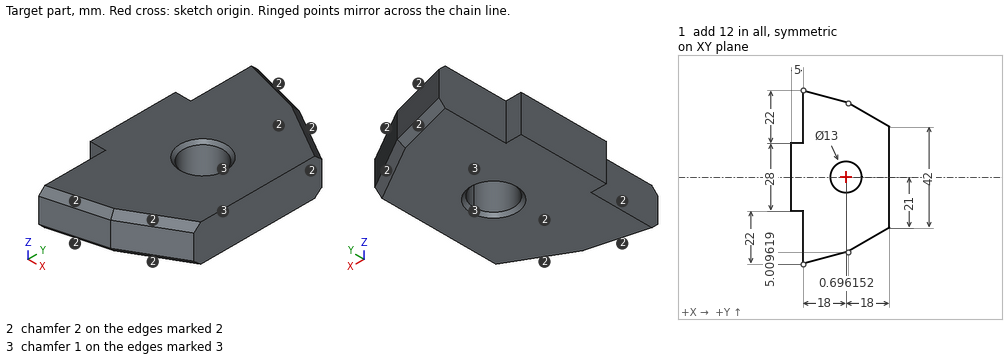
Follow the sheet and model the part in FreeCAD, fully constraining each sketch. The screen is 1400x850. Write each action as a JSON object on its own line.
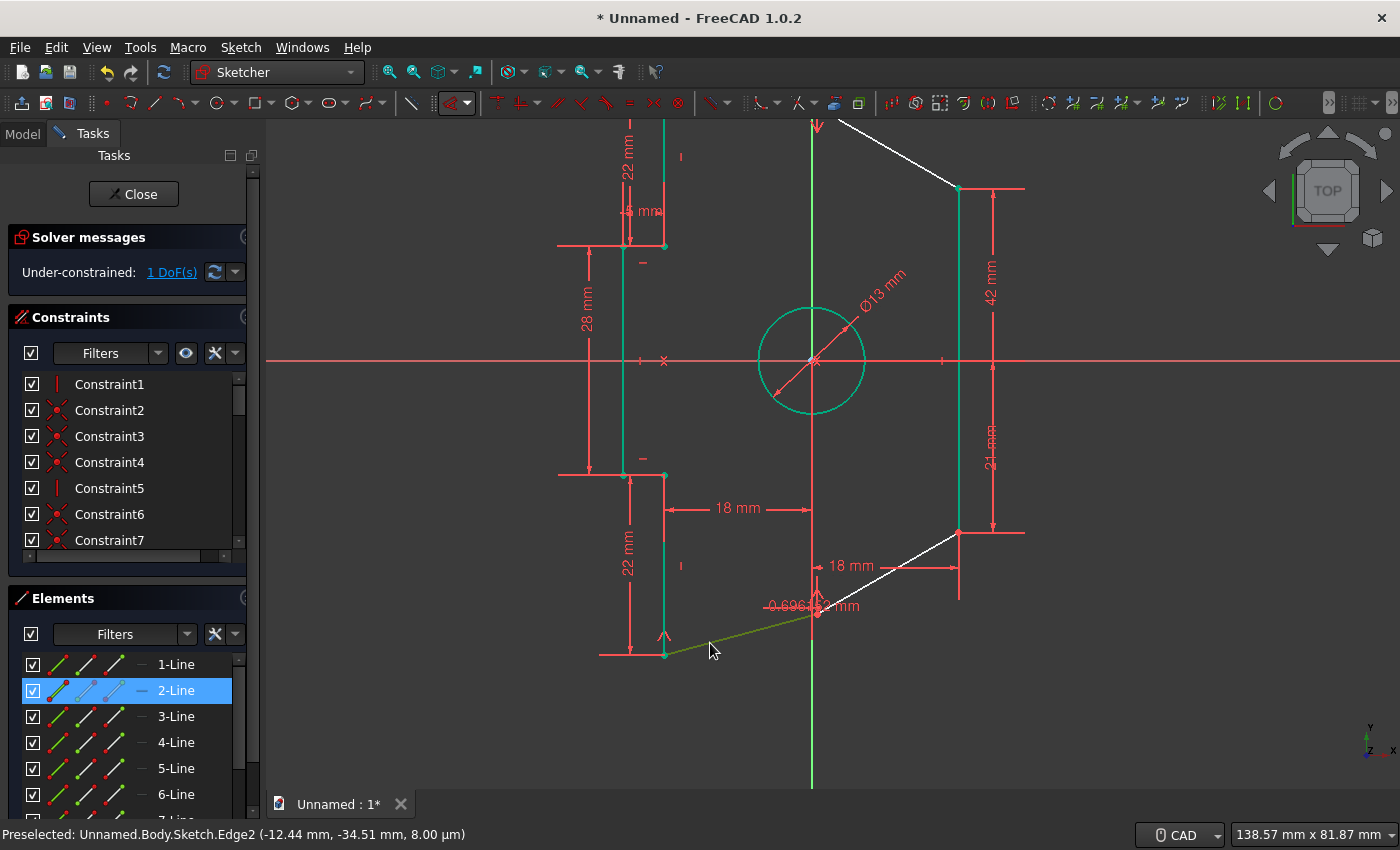
{"action": "left_click", "coordinate": [470, 104]}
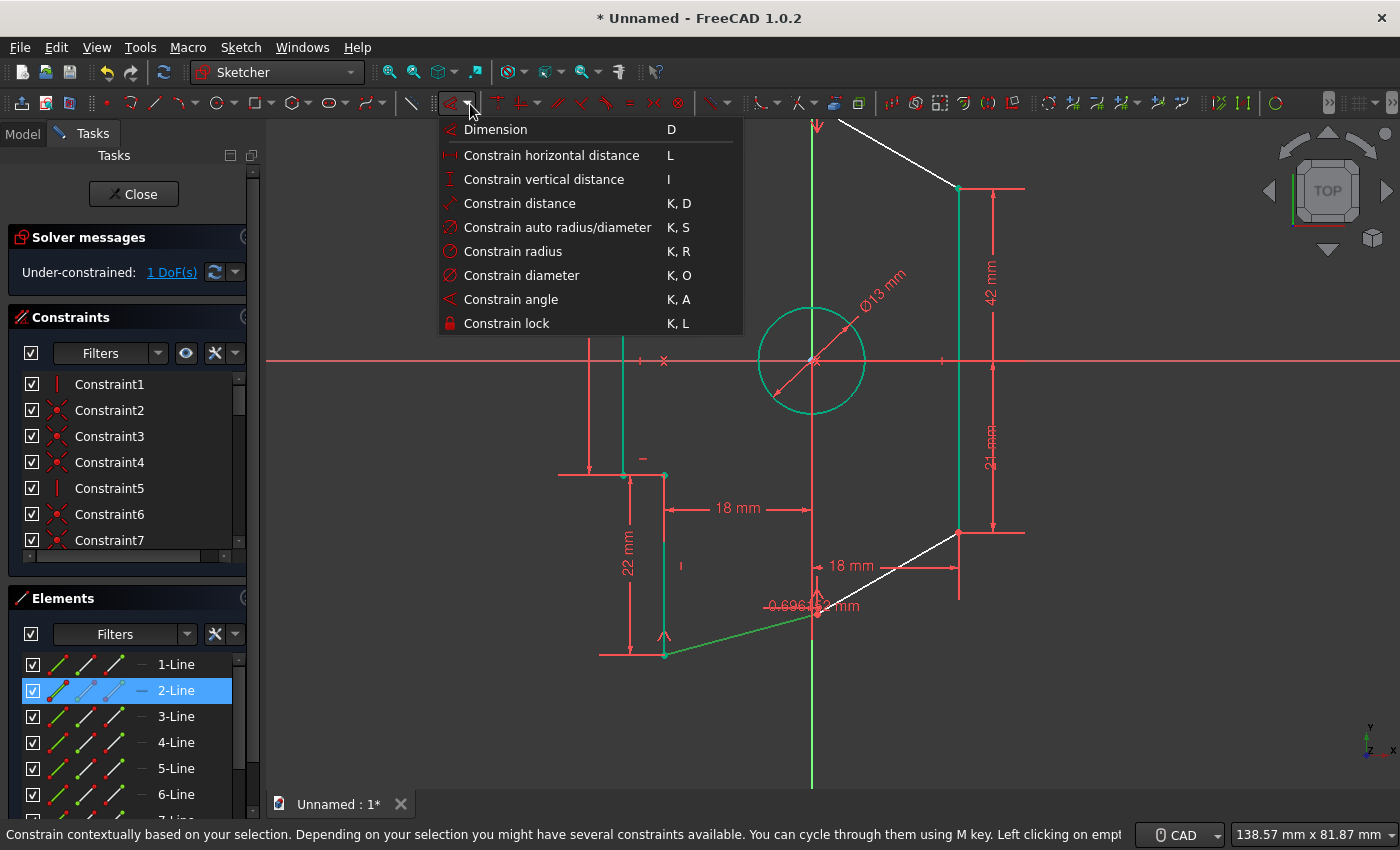
{"action": "left_click", "coordinate": [591, 179]}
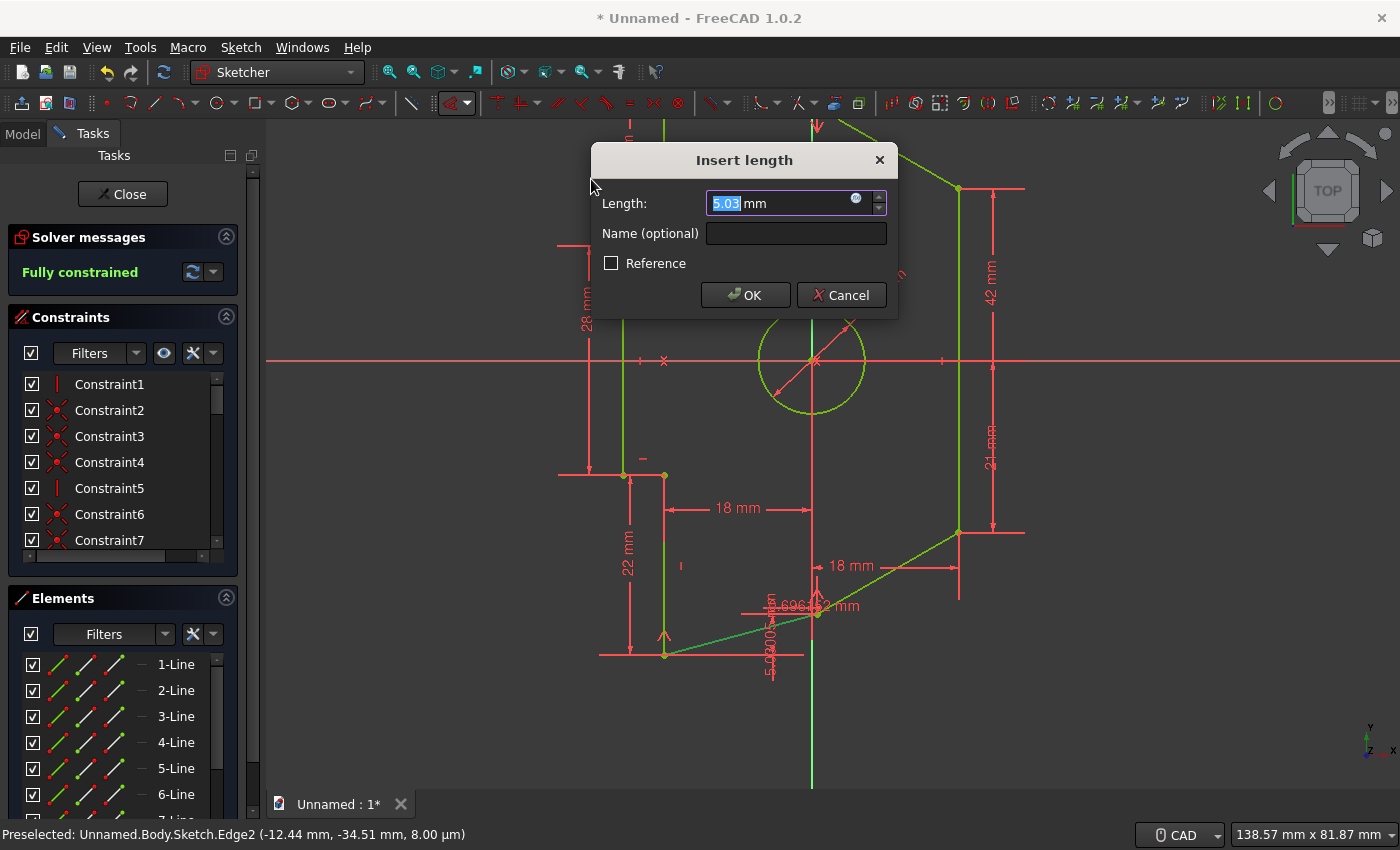
{"action": "type", "text": "5.009619"}
{"action": "key", "text": "Return"}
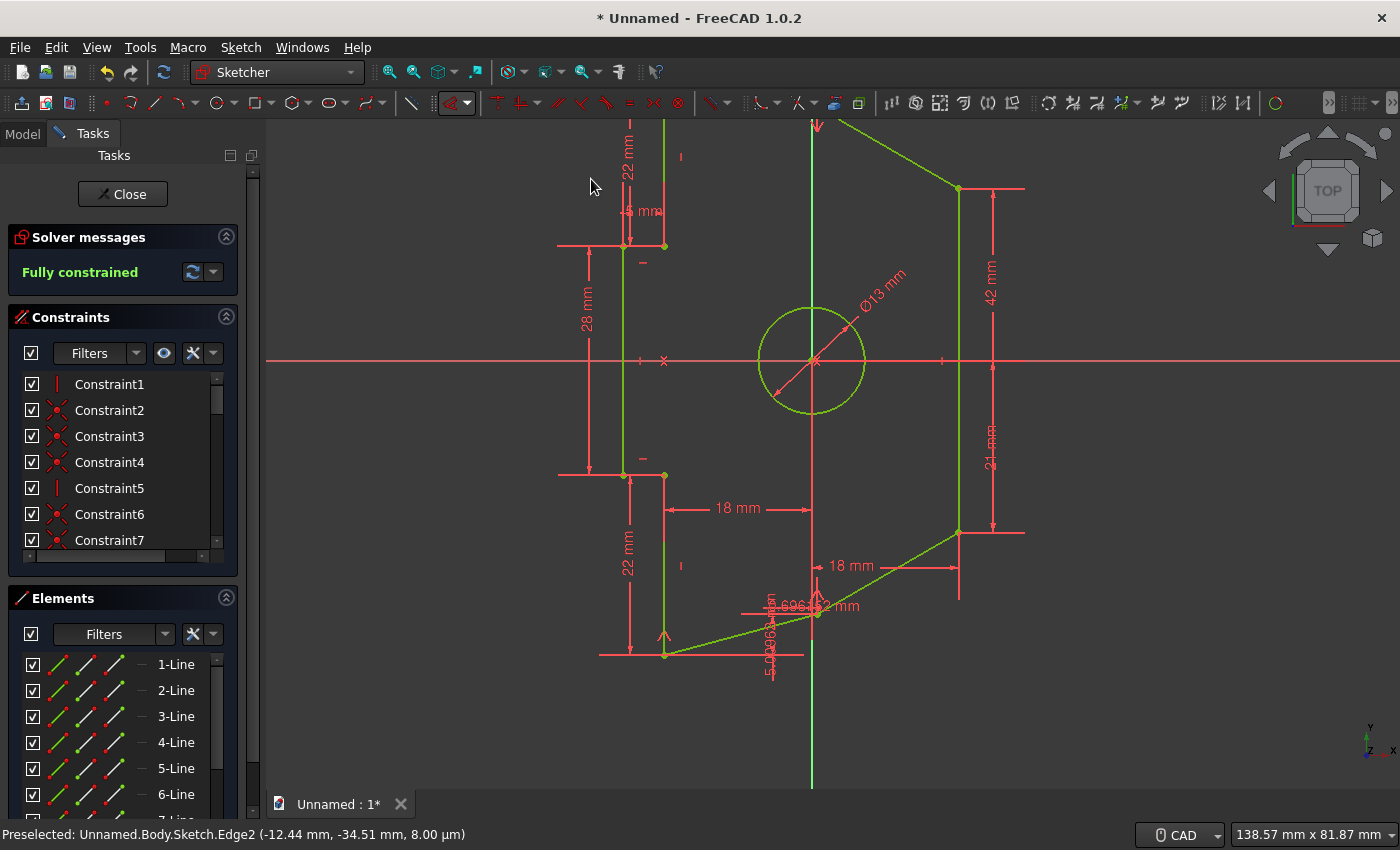
{"action": "left_click", "coordinate": [123, 194]}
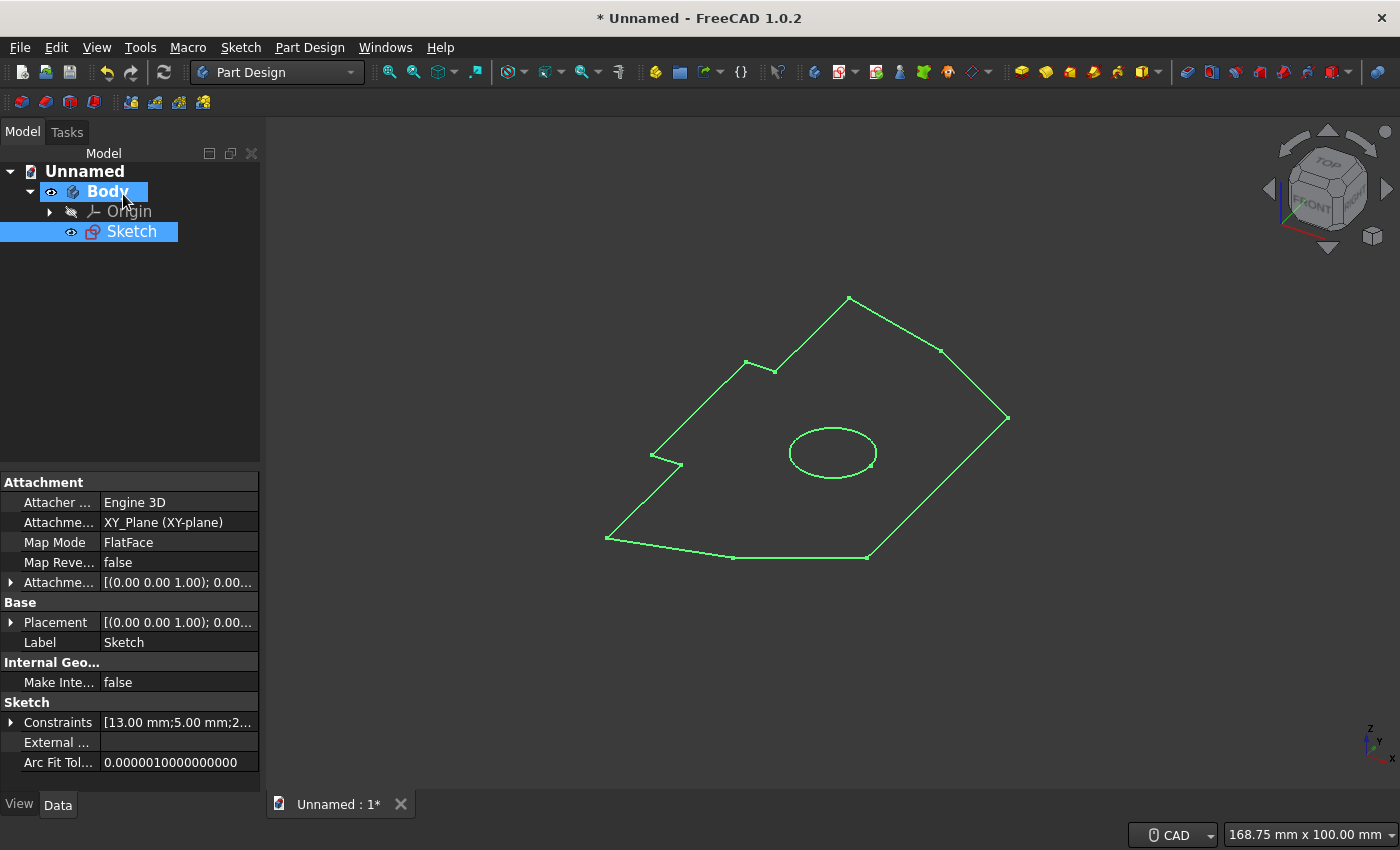
{"action": "left_click", "coordinate": [1022, 72]}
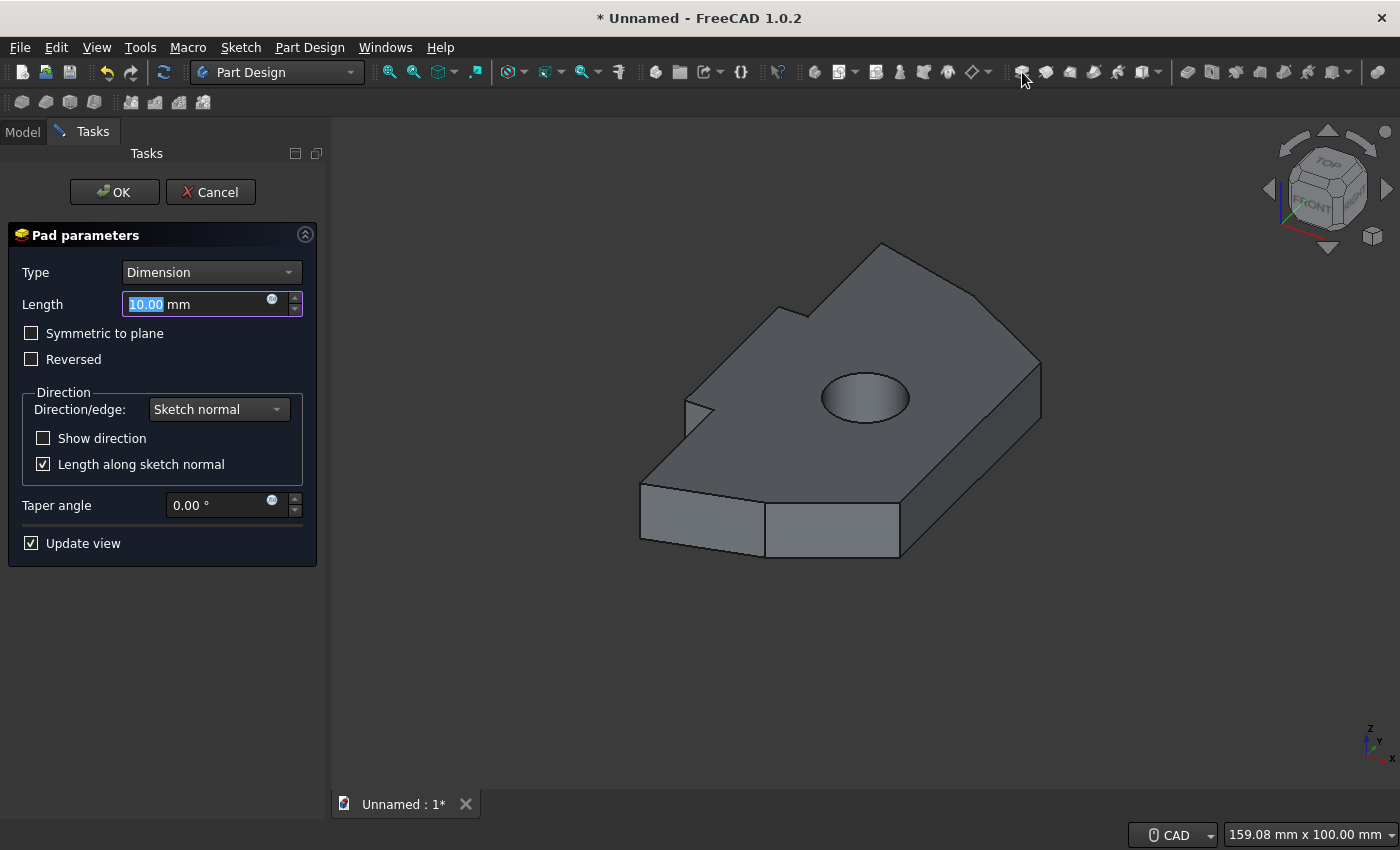
{"action": "type", "text": "12"}
{"action": "key", "text": "Tab"}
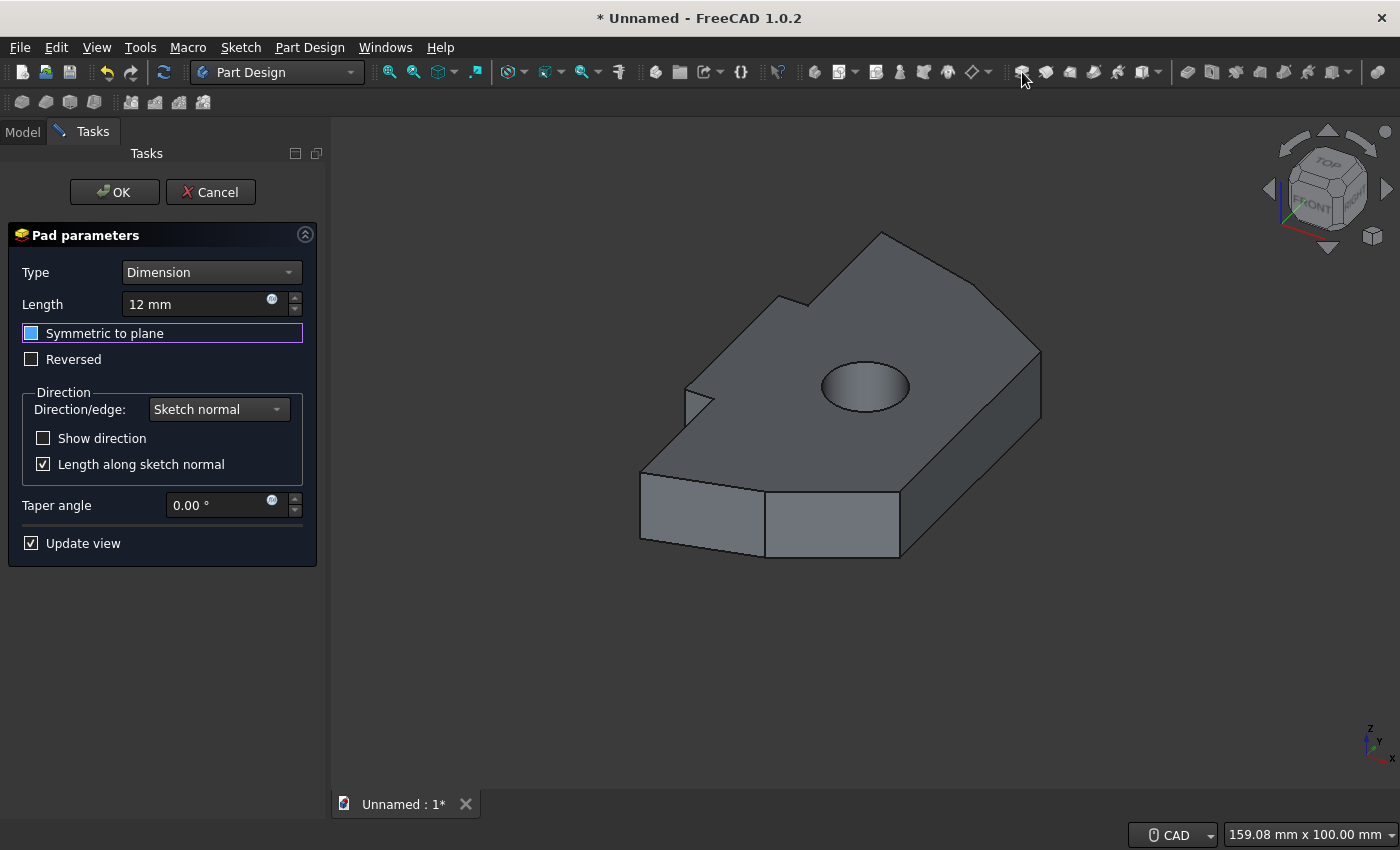
{"action": "left_click", "coordinate": [30, 333]}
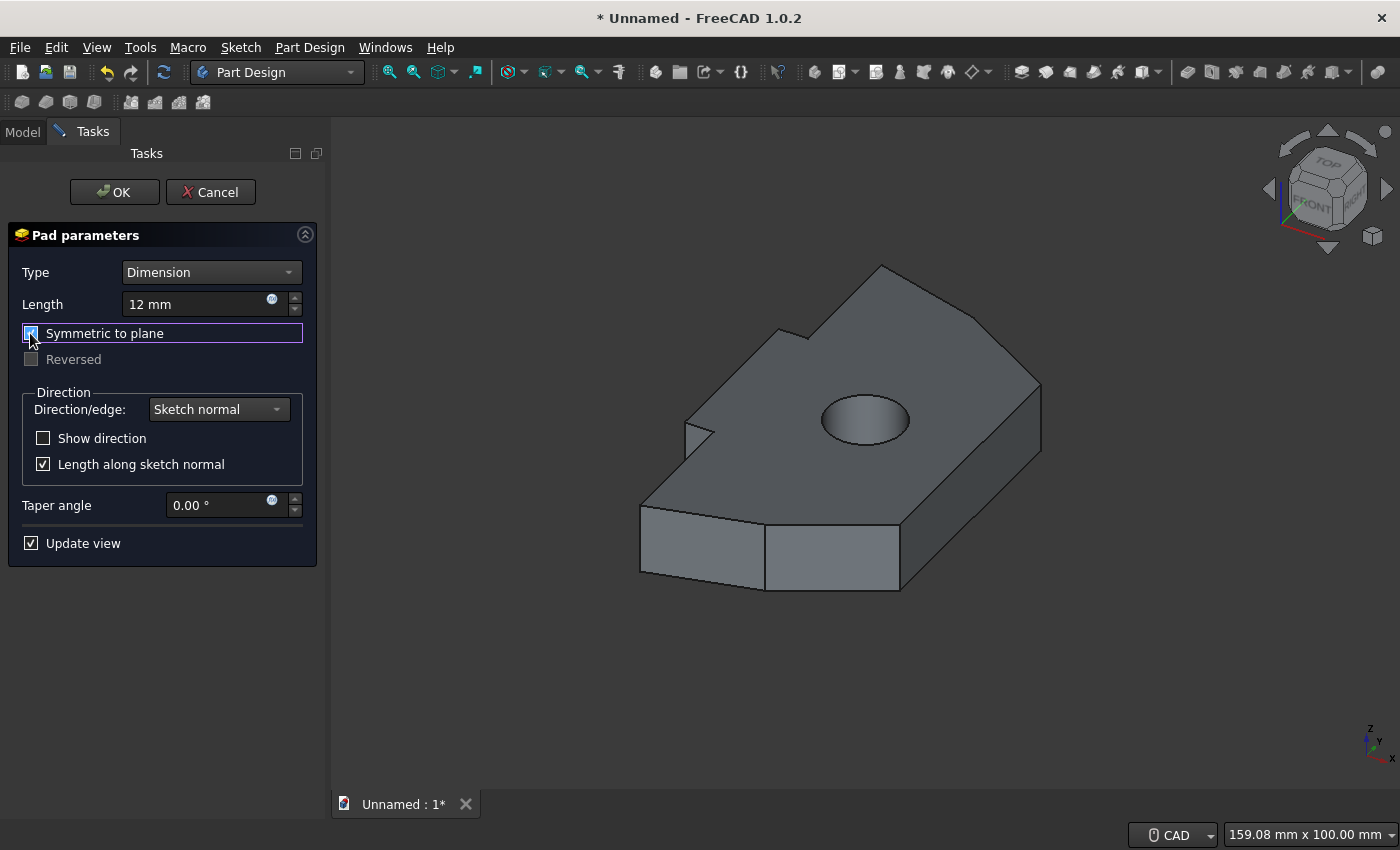
{"action": "left_click", "coordinate": [115, 192]}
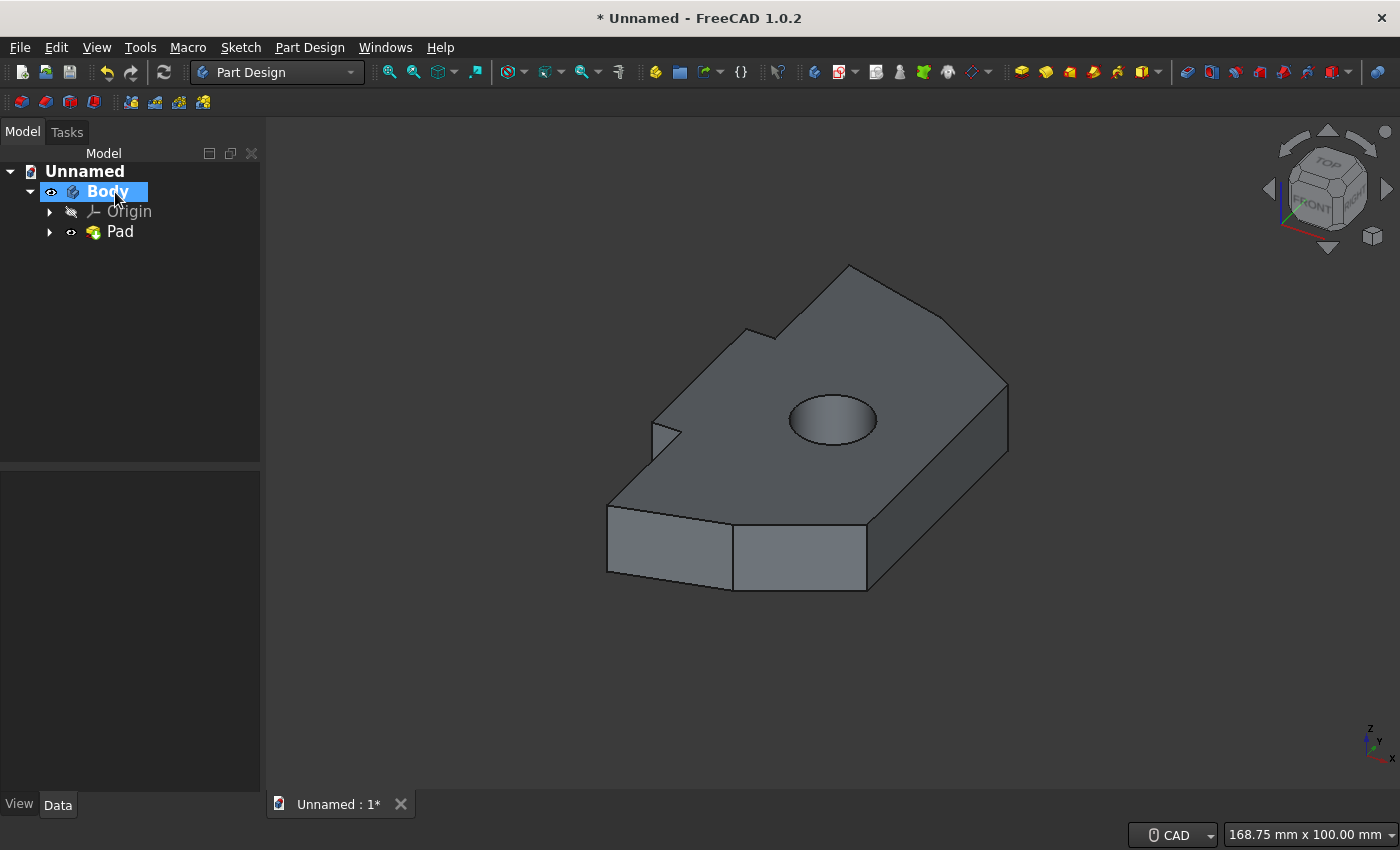
{"action": "left_click", "coordinate": [800, 524]}